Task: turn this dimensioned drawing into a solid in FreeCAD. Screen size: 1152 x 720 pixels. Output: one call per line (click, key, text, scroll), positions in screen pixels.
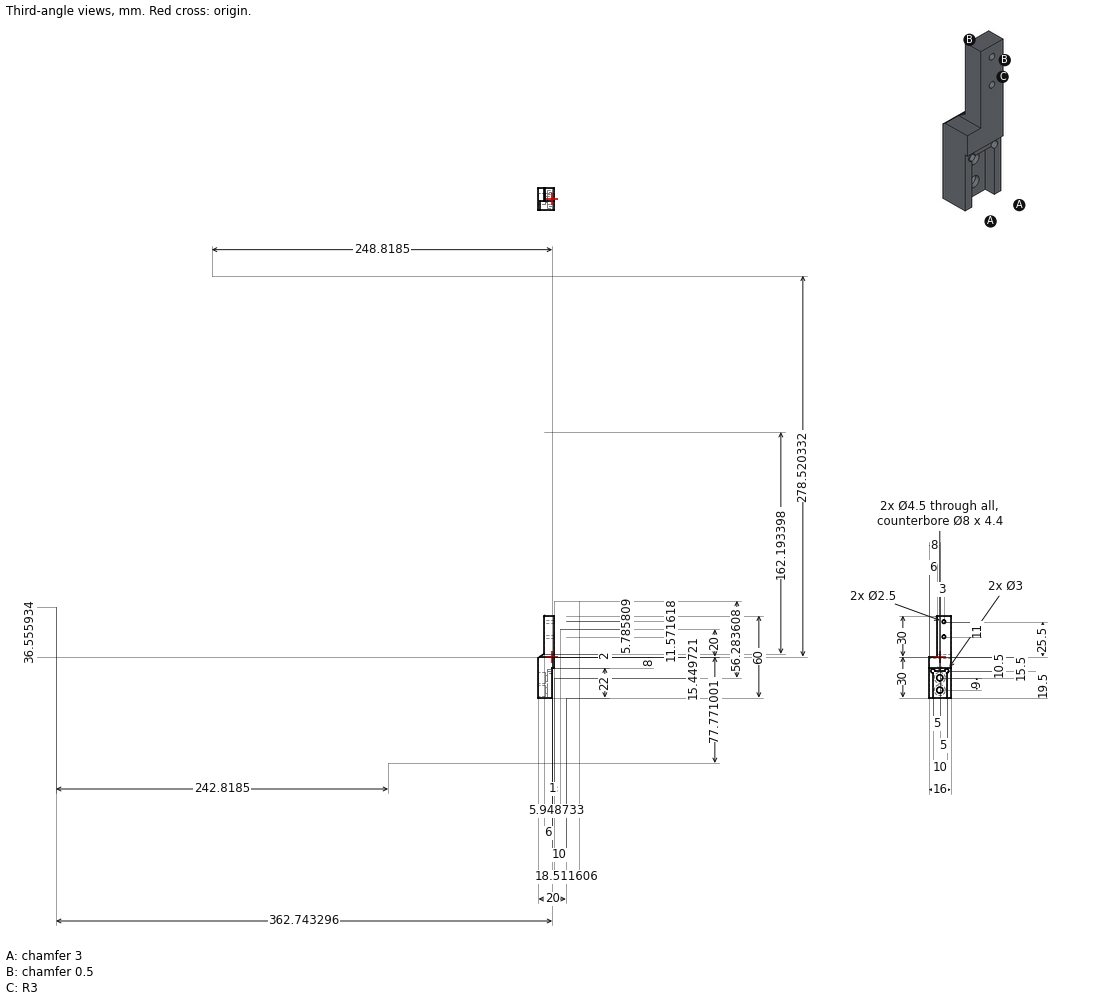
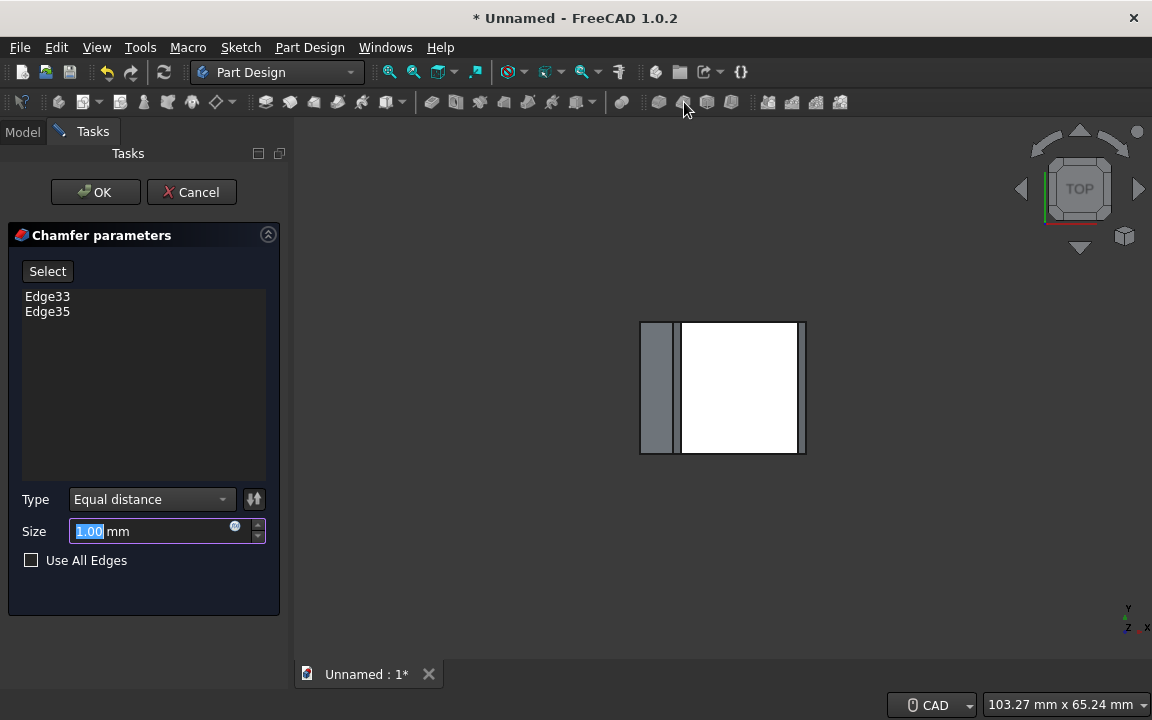
text(0.5)
key(Tab)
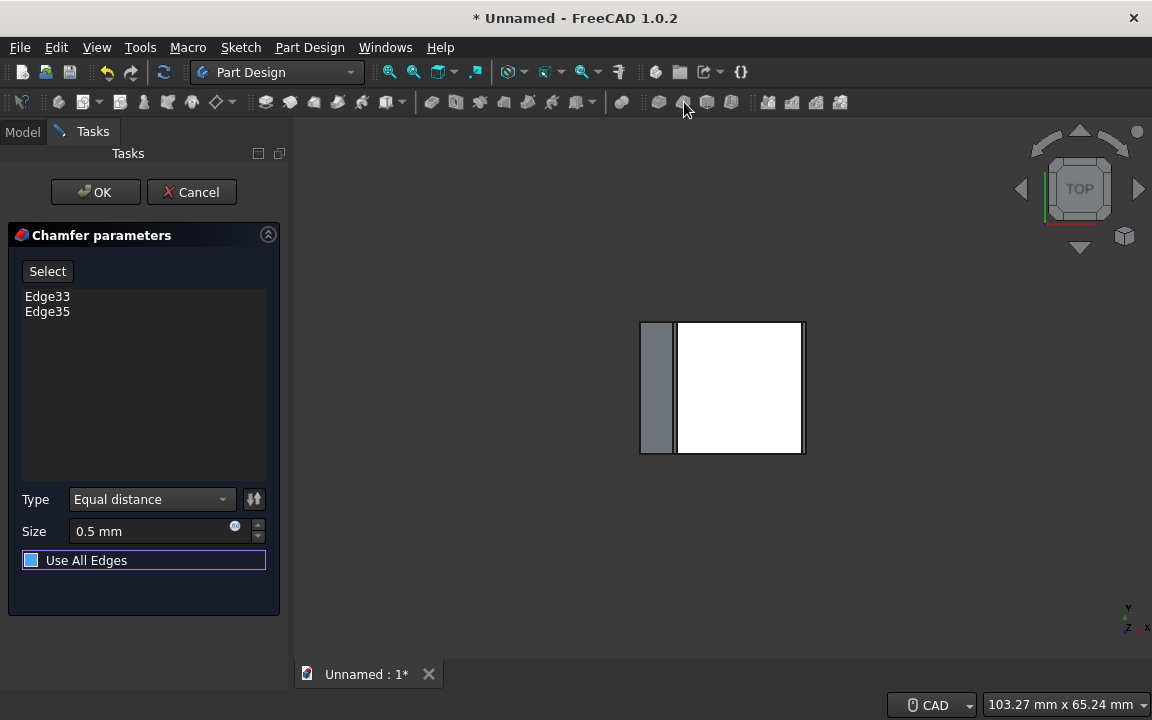
click(96, 192)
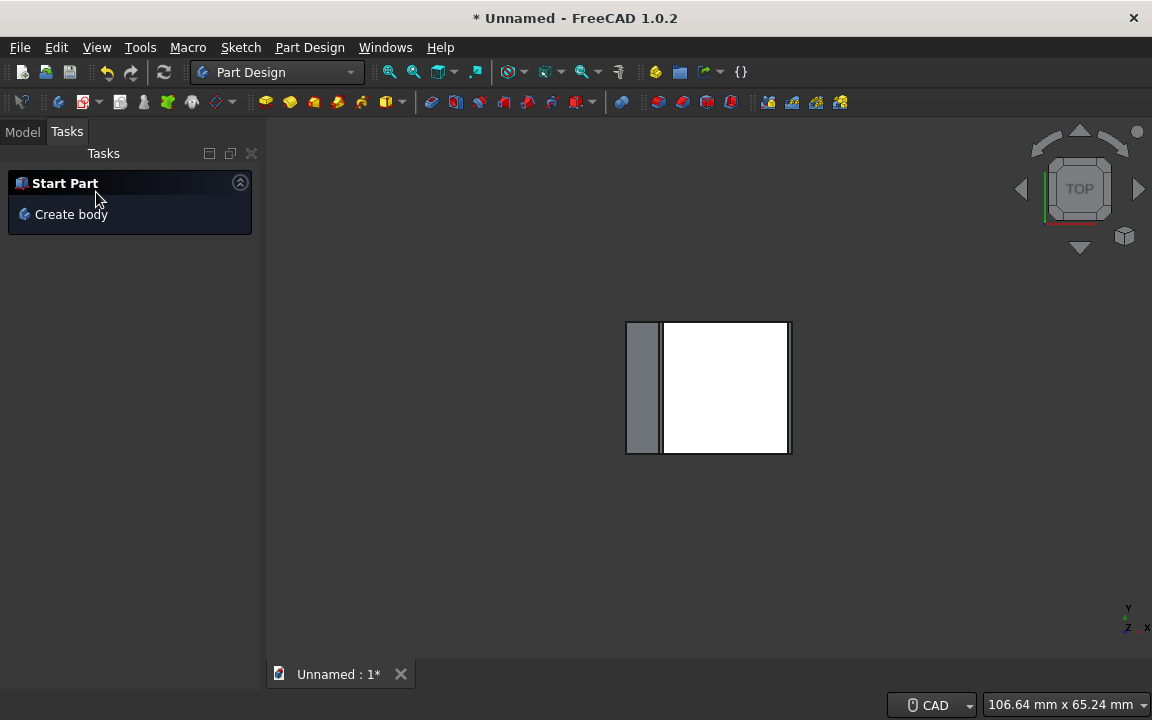
key(v)
key(f)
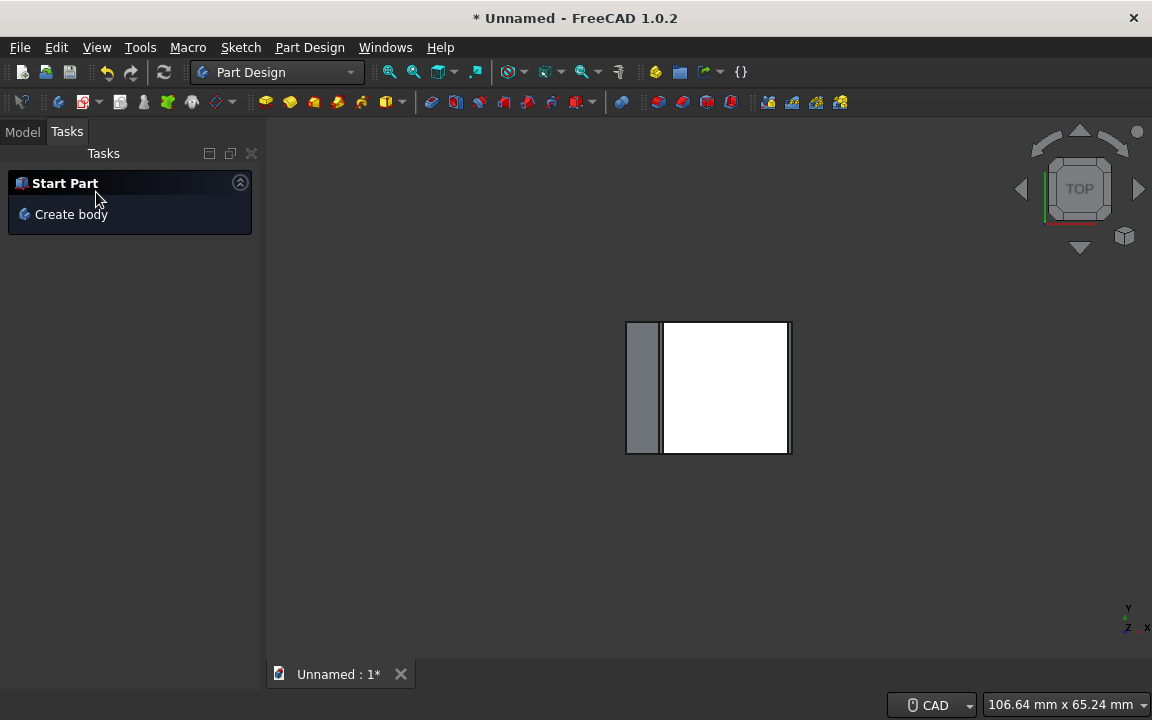
key(0)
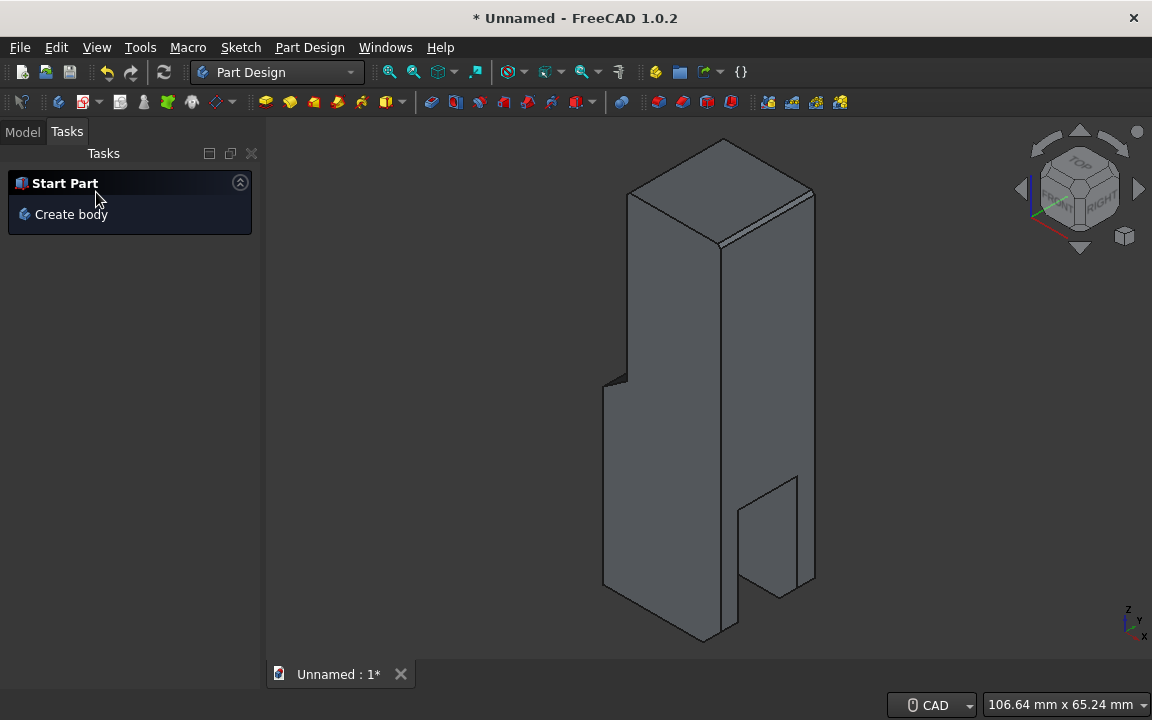
click(768, 303)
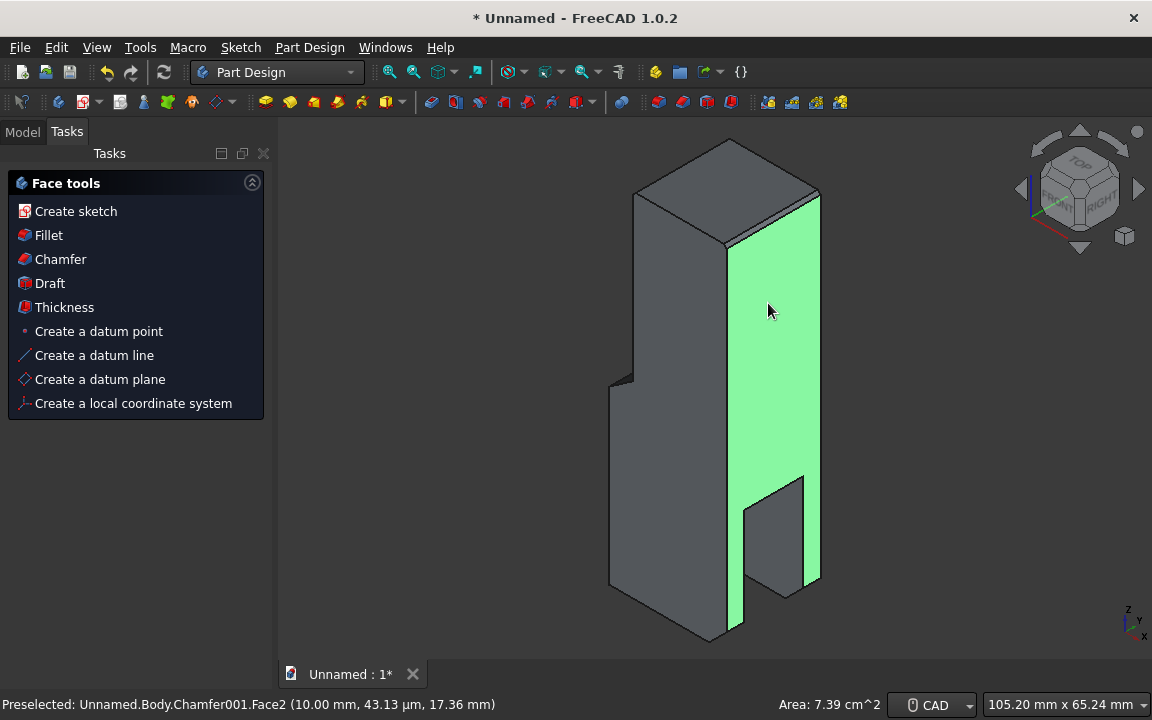
click(84, 102)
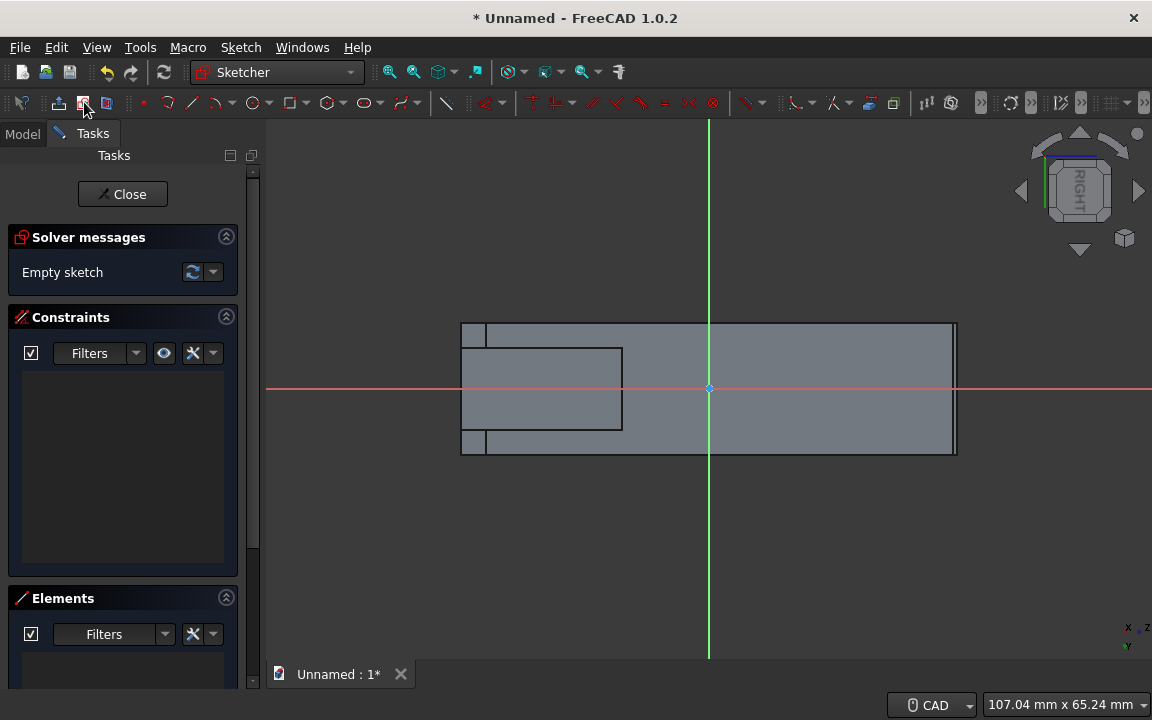
scroll(667, 389, up, 6)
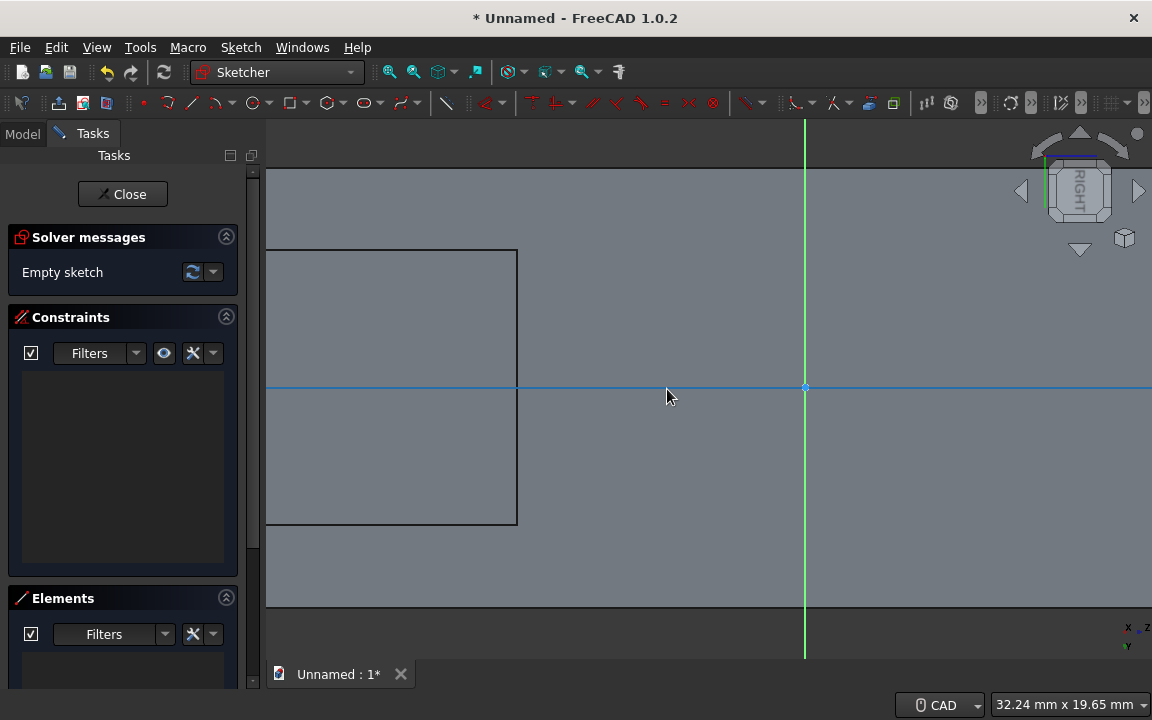
click(254, 104)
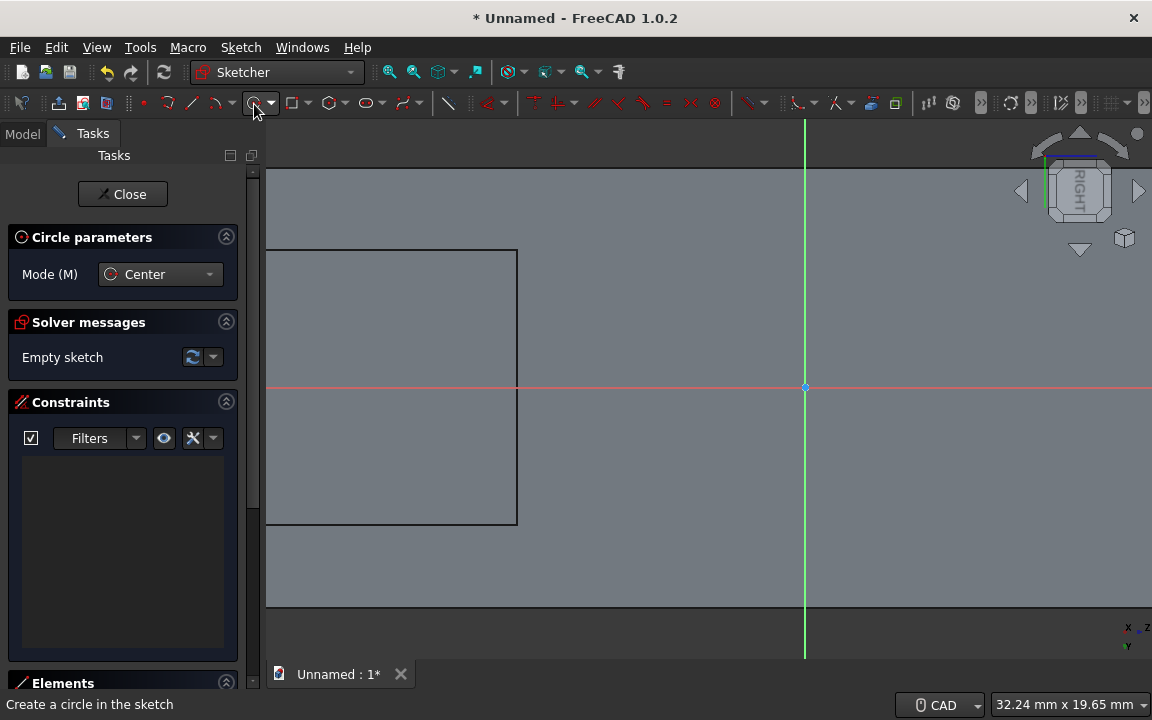
click(517, 525)
click(546, 496)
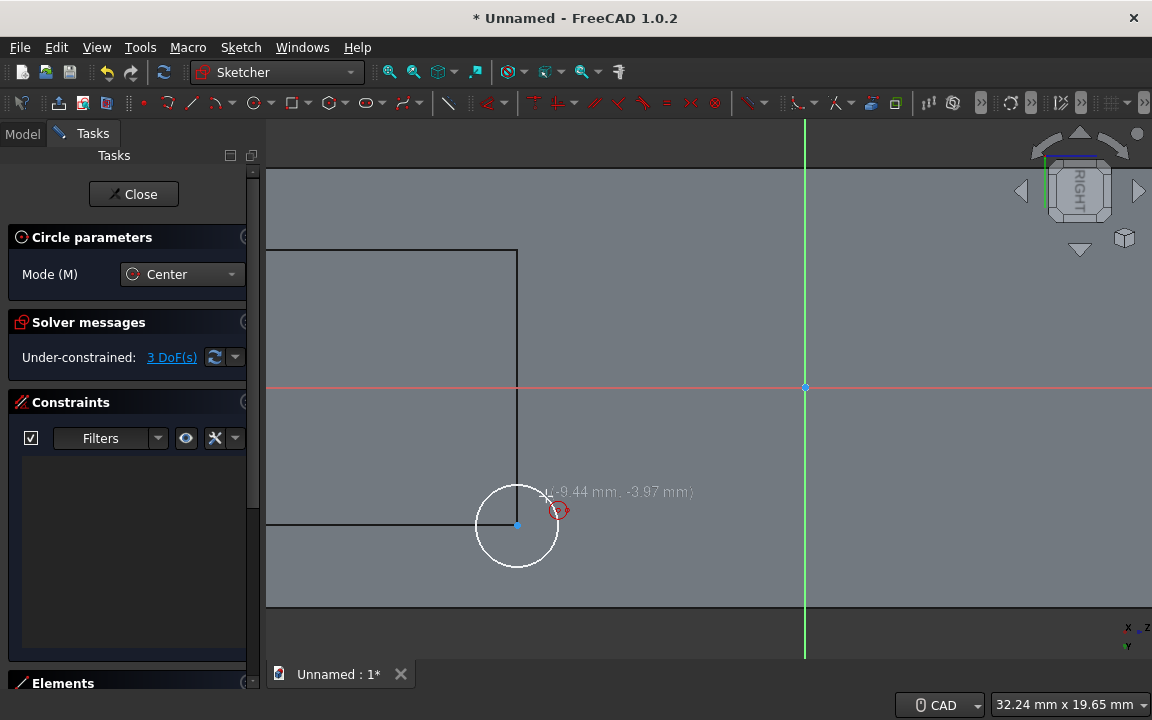
click(517, 250)
click(546, 221)
key(Escape)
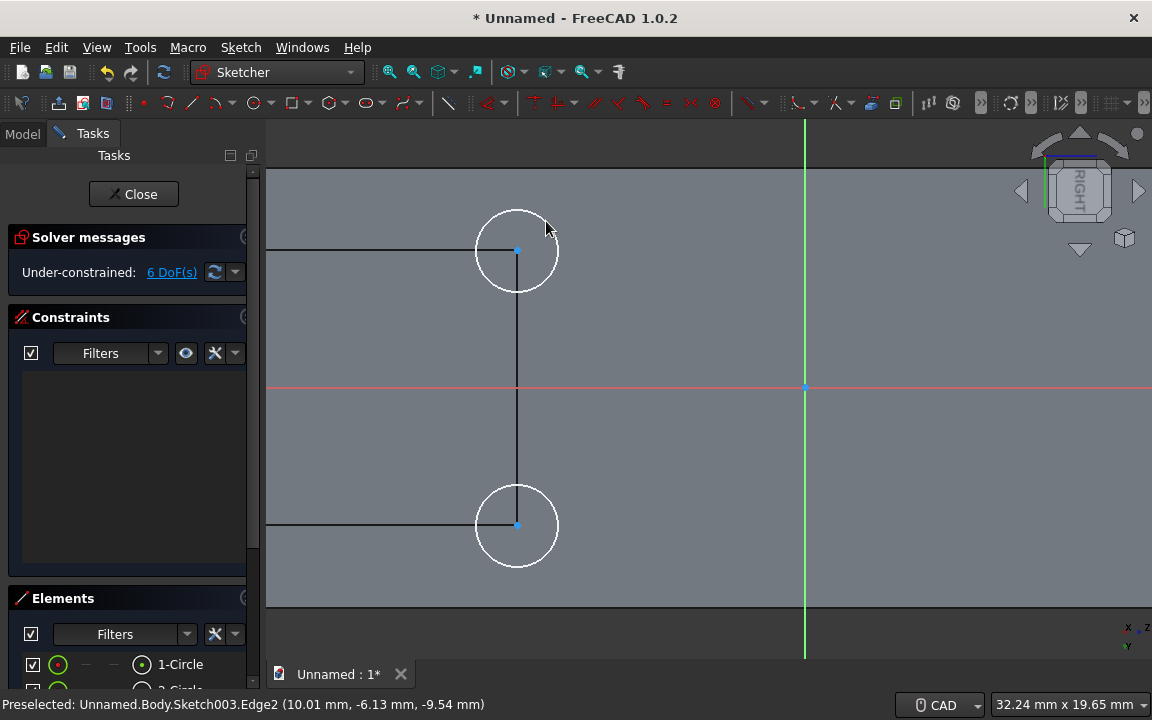
click(546, 497)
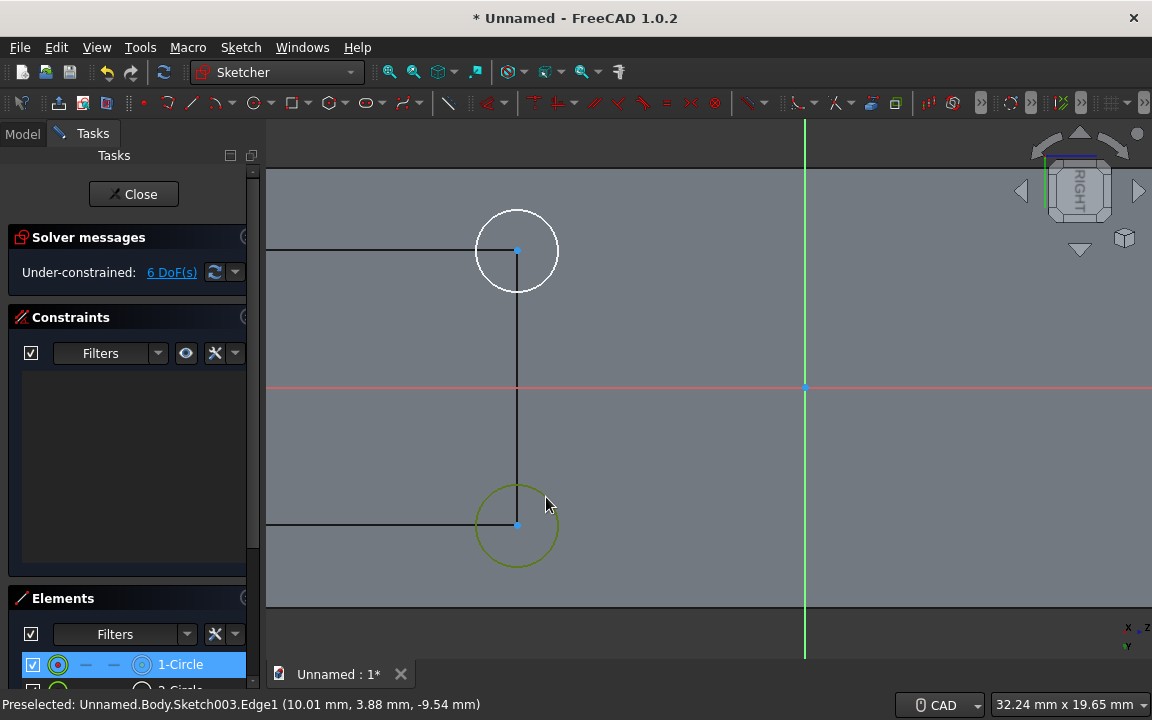
click(546, 222)